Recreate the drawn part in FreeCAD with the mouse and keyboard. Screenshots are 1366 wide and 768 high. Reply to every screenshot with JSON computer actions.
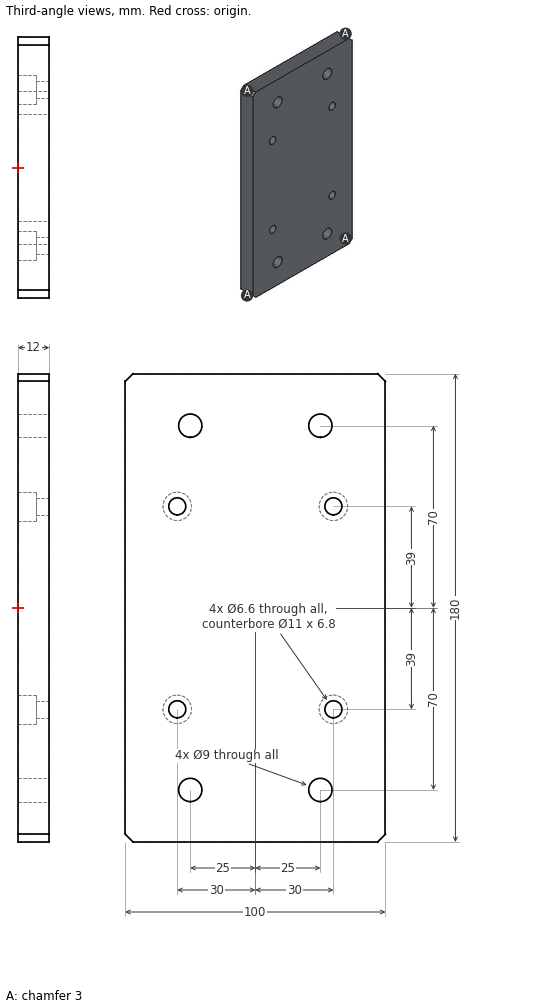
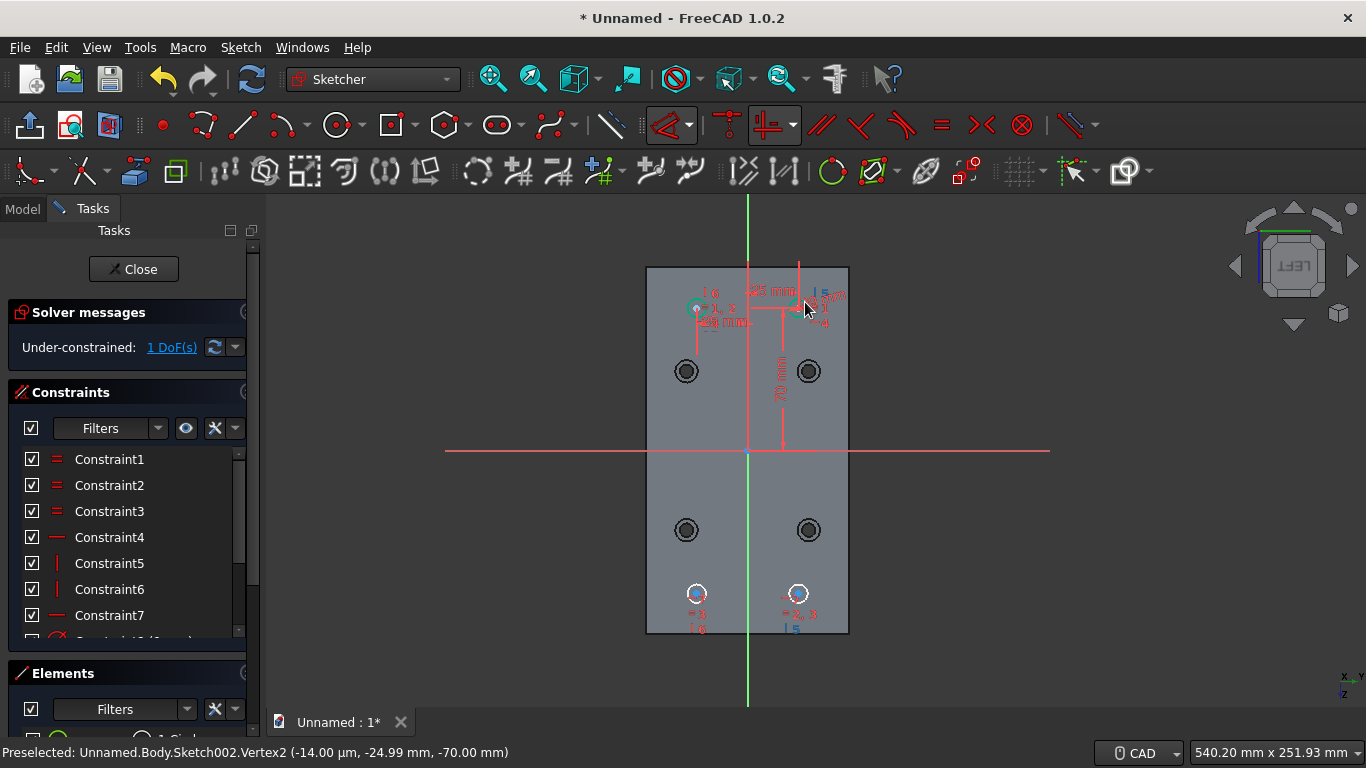
{"action": "left_click", "coordinate": [799, 594]}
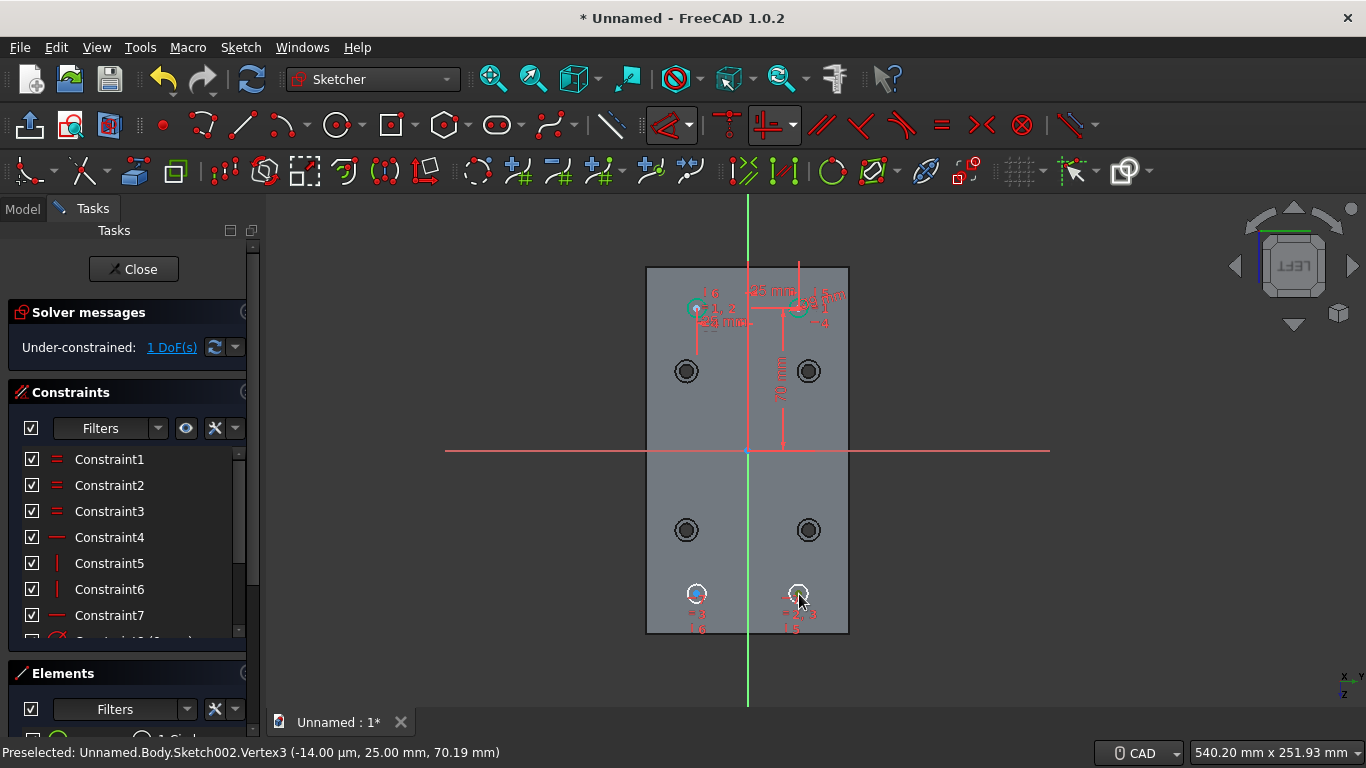
{"action": "left_click", "coordinate": [692, 126]}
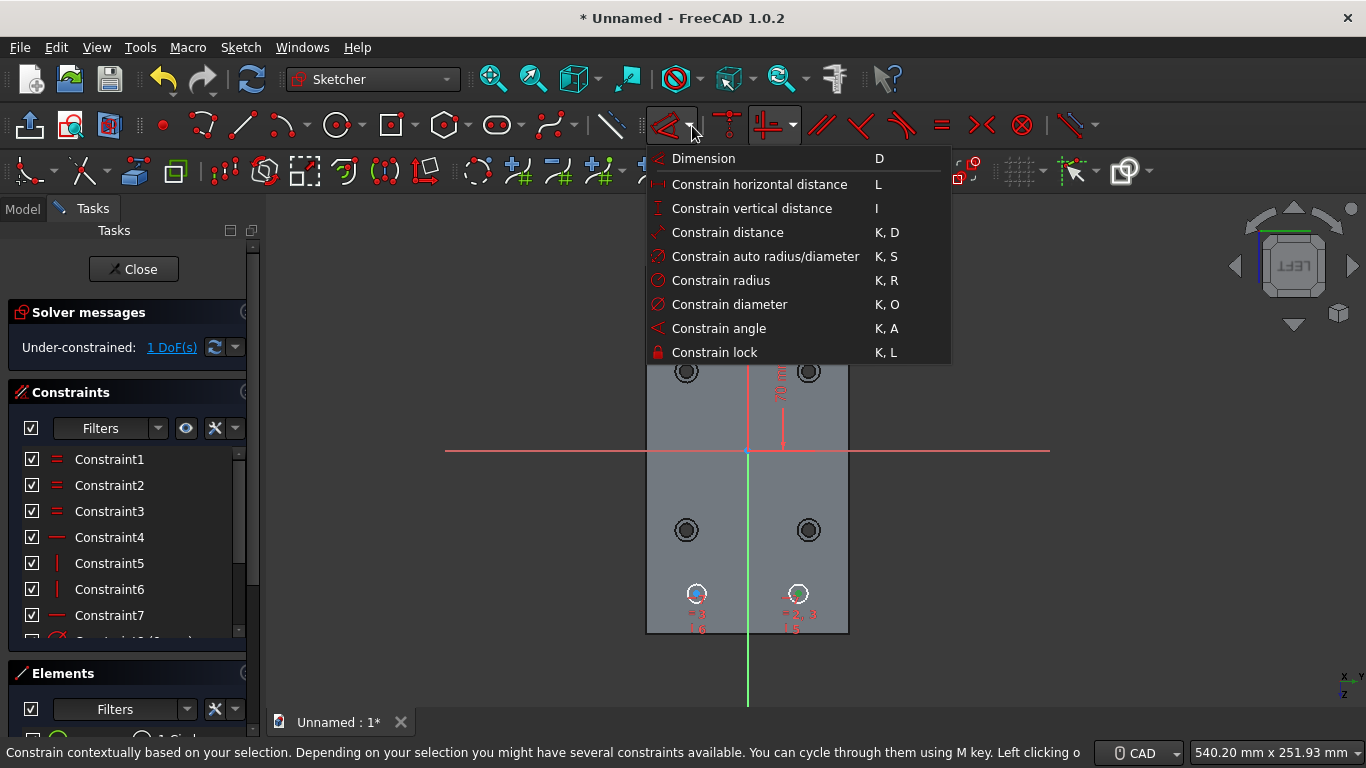
{"action": "left_click", "coordinate": [799, 208]}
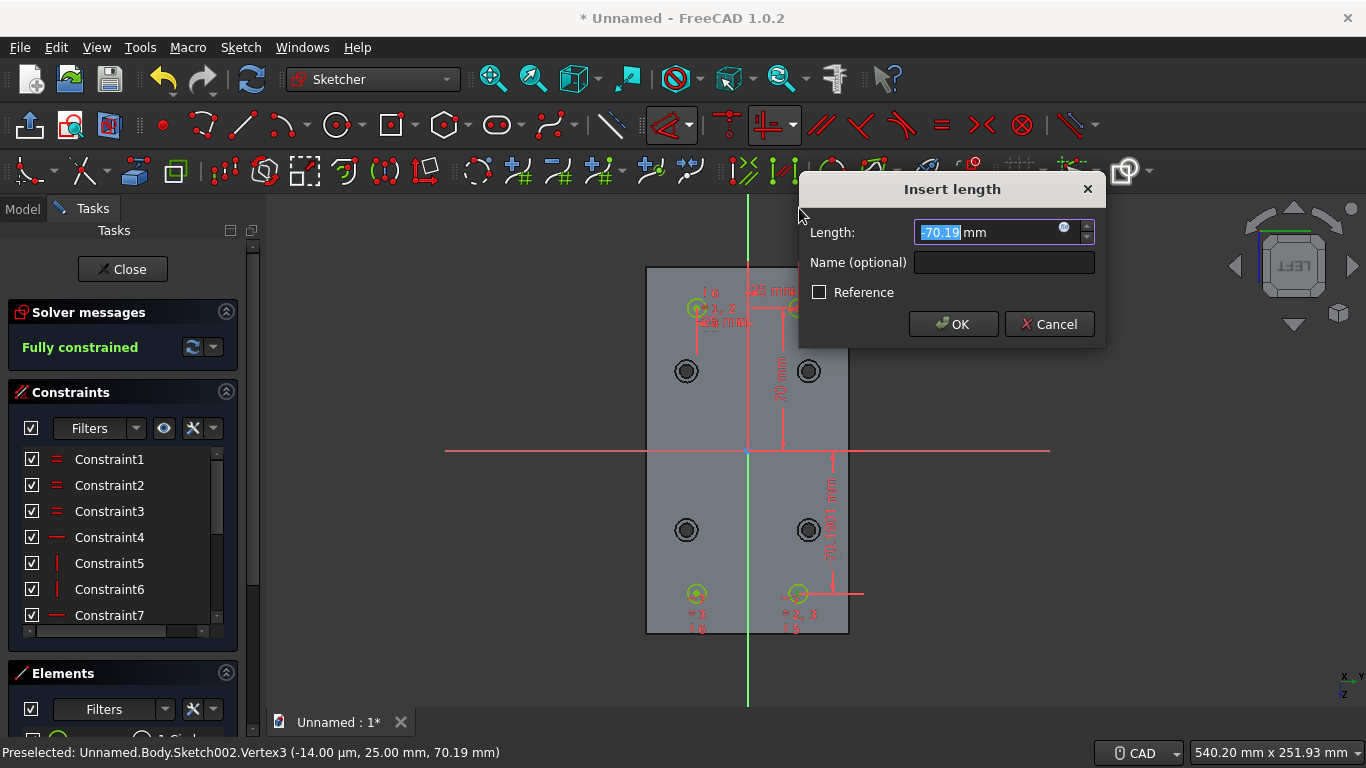
{"action": "type", "text": "-70"}
{"action": "key", "text": "Return"}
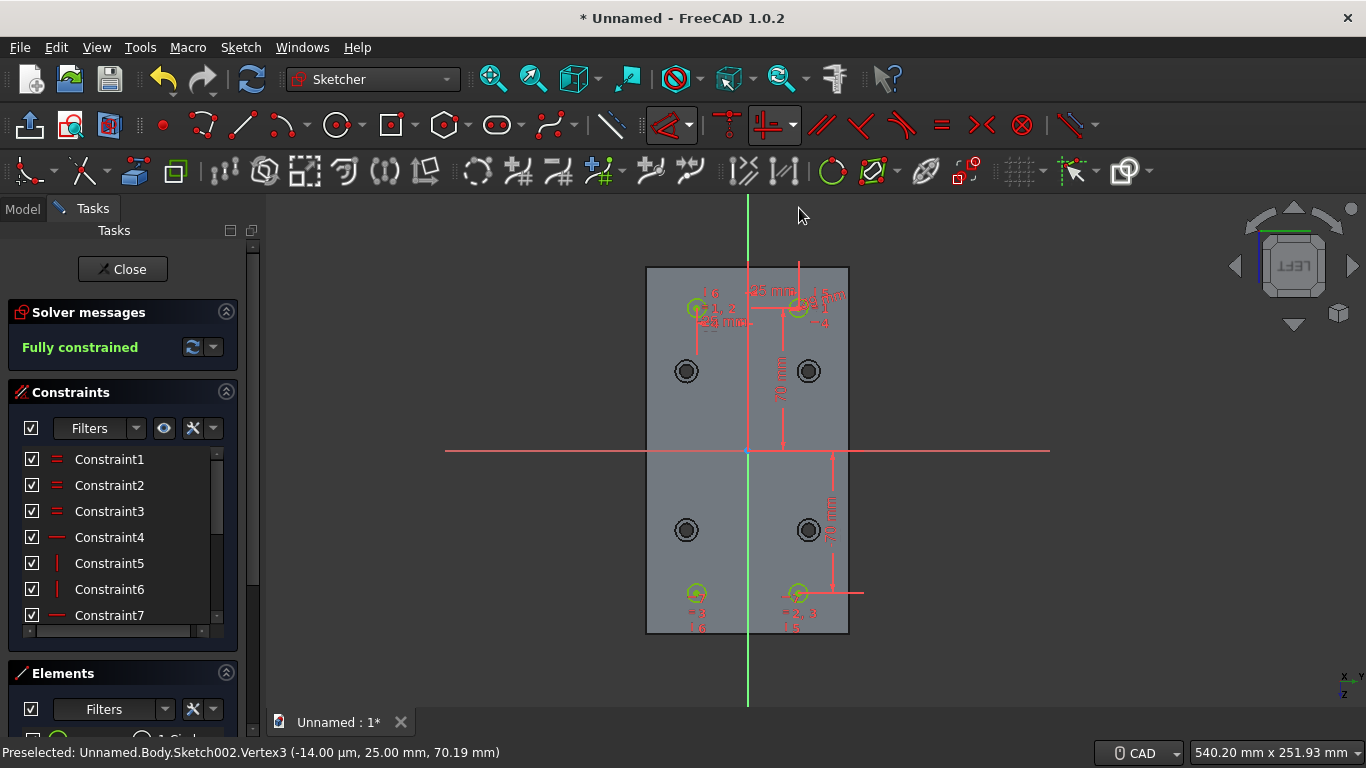
{"action": "left_click", "coordinate": [123, 269]}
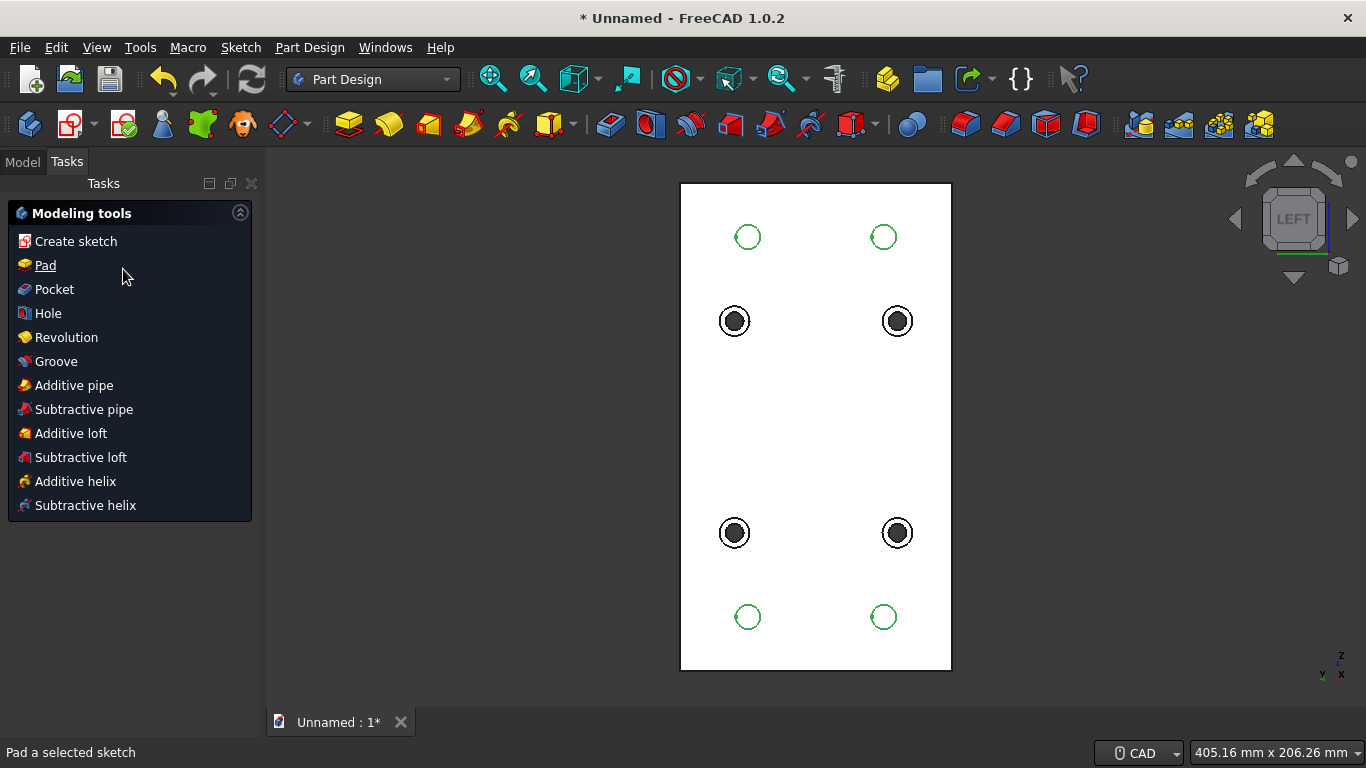
{"action": "left_click", "coordinate": [652, 124]}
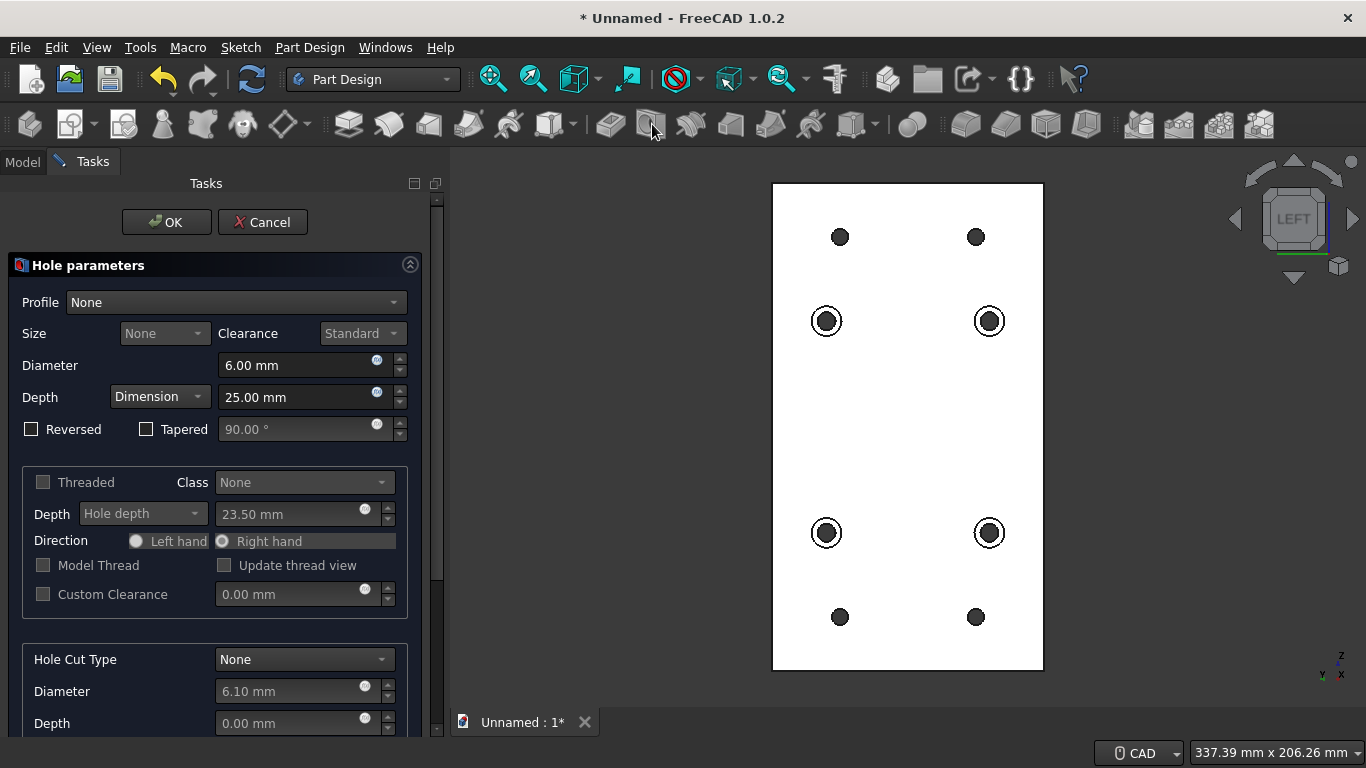
{"action": "triple_click", "coordinate": [305, 365]}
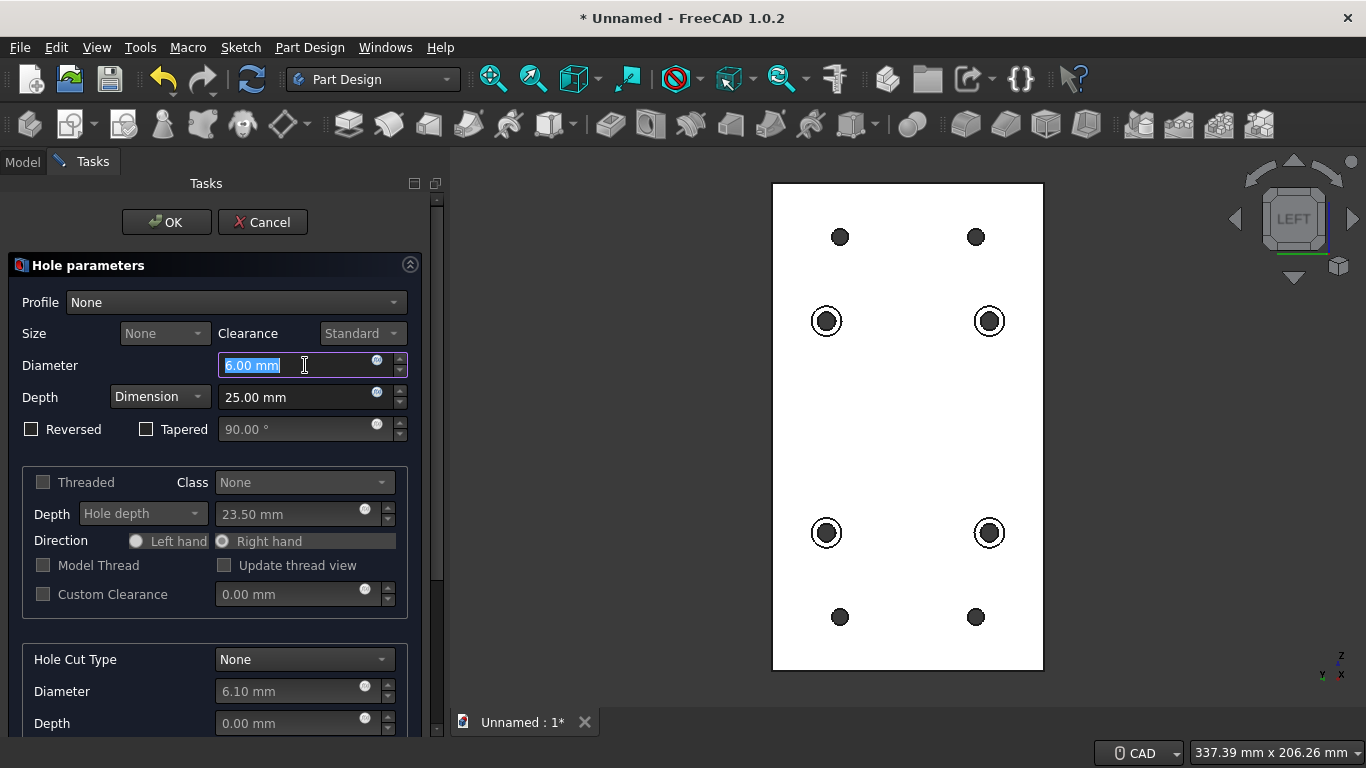
{"action": "type", "text": "9"}
{"action": "key", "text": "Tab"}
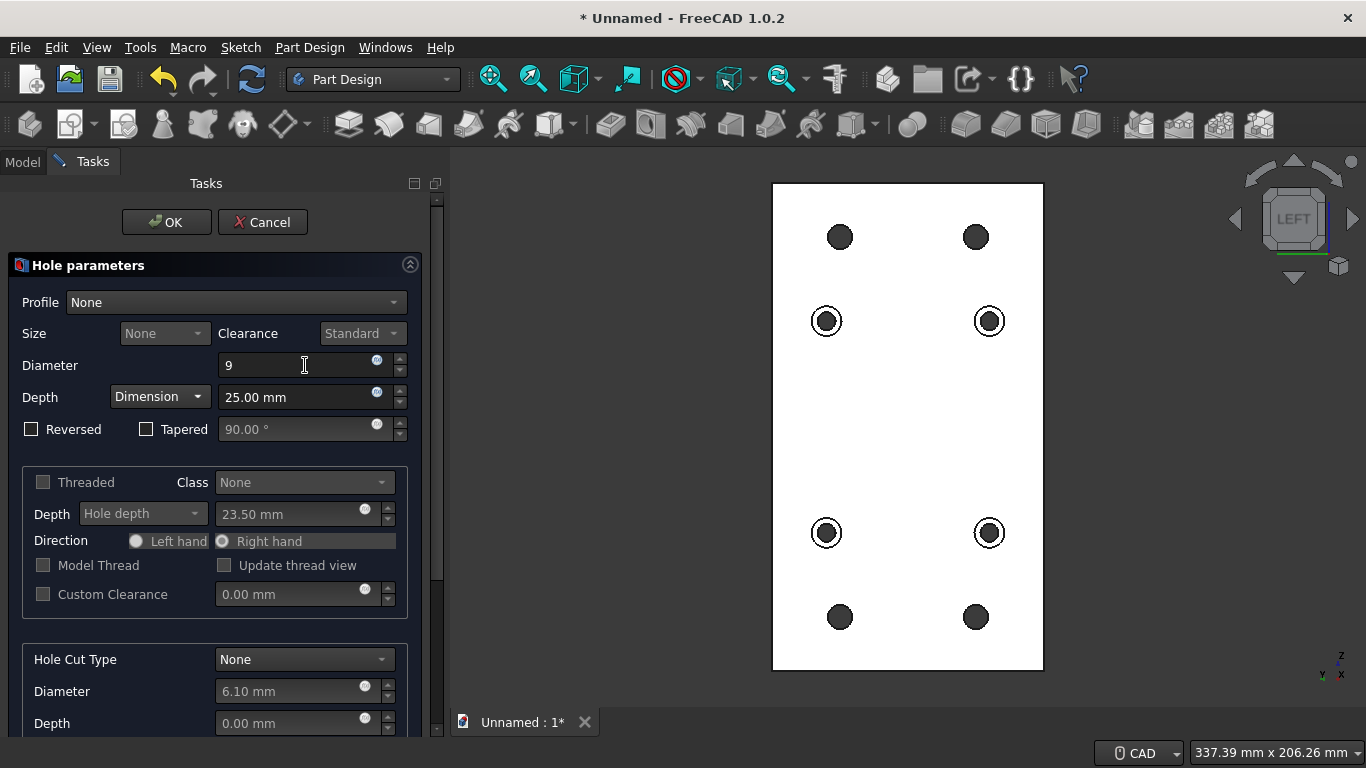
{"action": "left_click", "coordinate": [161, 396]}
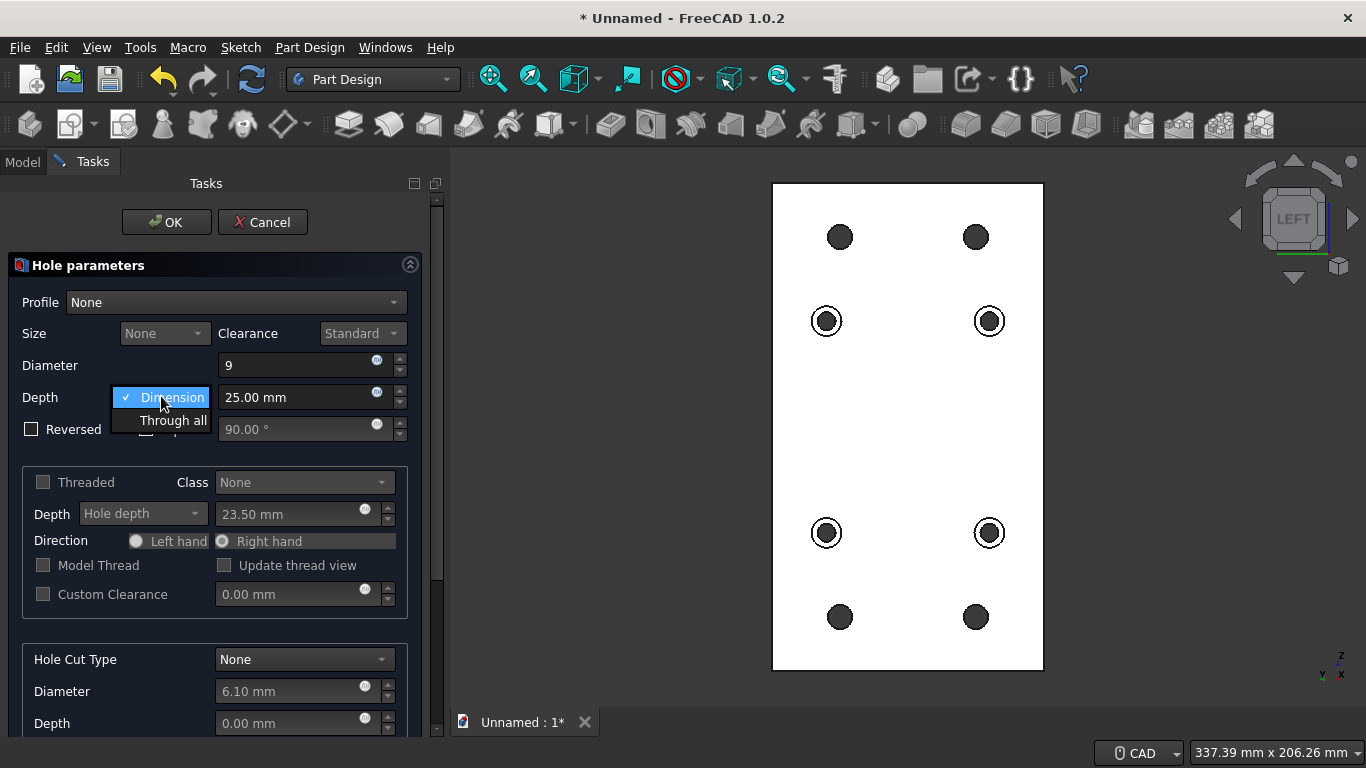
{"action": "left_click", "coordinate": [160, 420]}